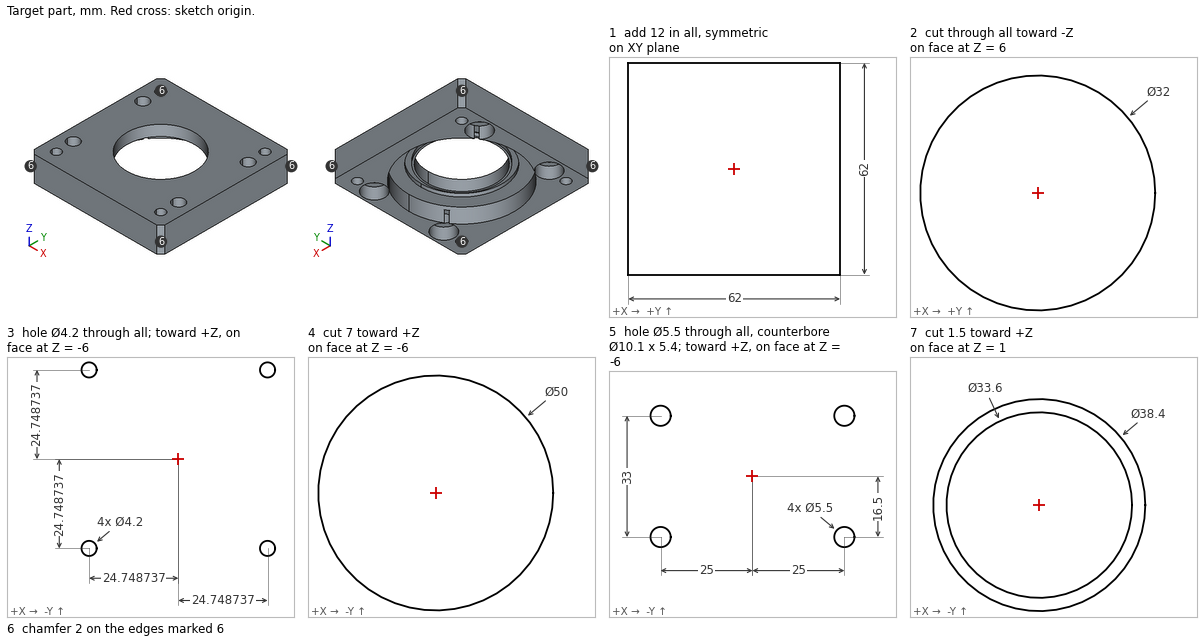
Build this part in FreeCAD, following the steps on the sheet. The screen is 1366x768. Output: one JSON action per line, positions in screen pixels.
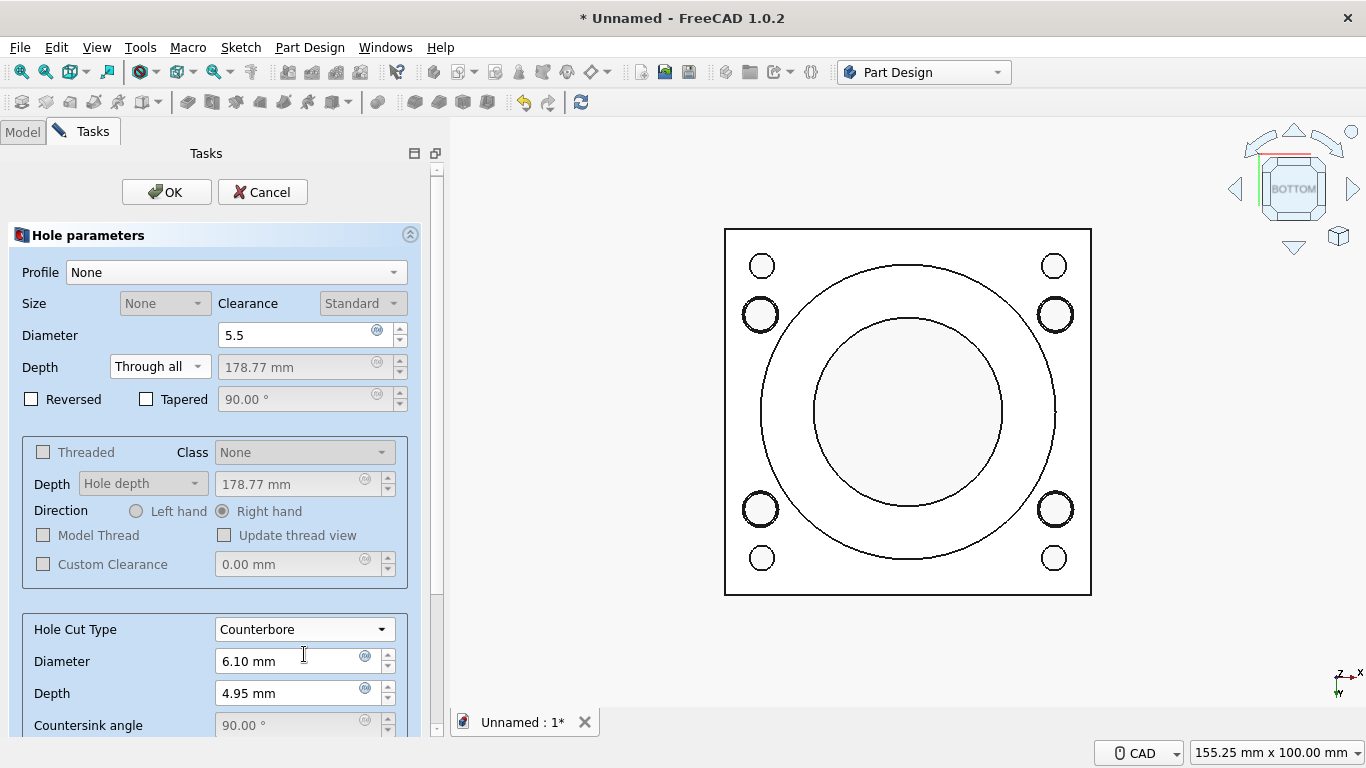
{"action": "triple_click", "coordinate": [298, 661]}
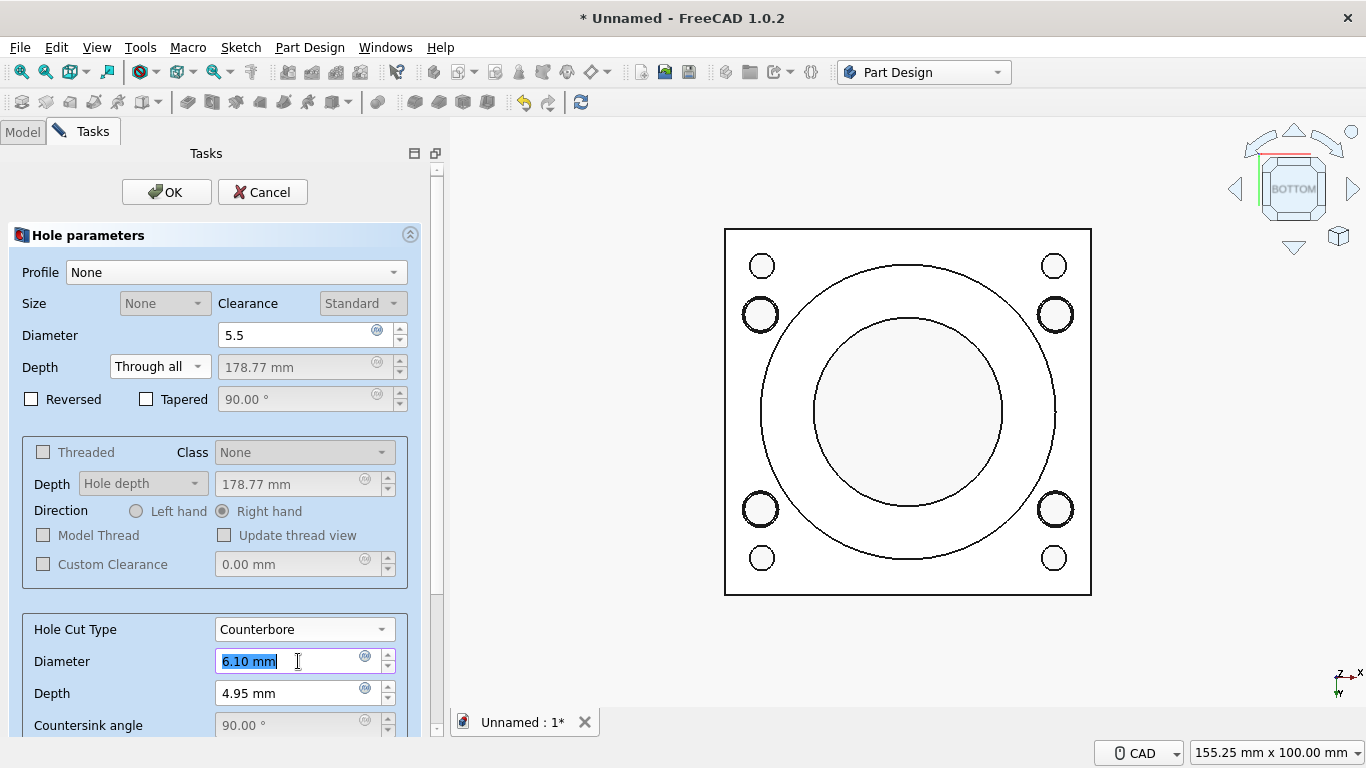
{"action": "type", "text": "10.1"}
{"action": "key", "text": "Tab"}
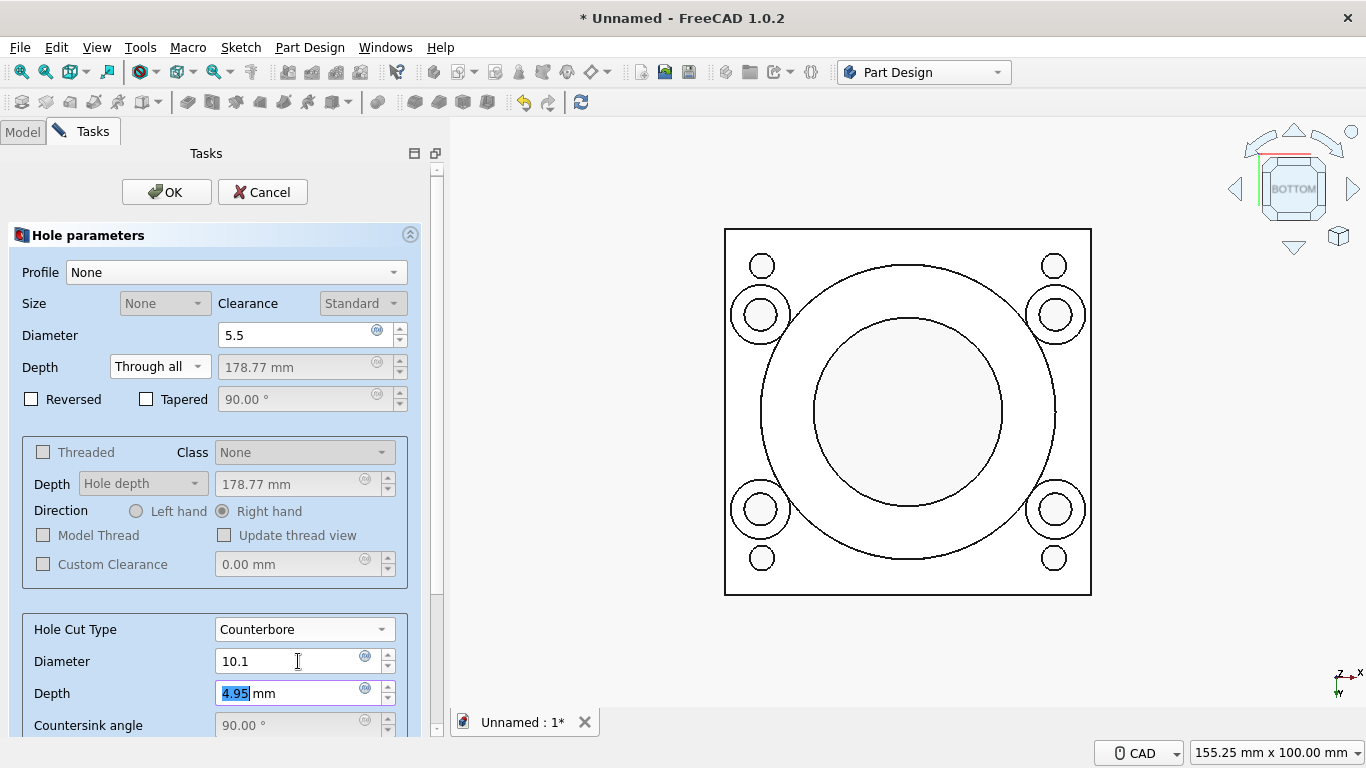
{"action": "type", "text": "5.4"}
{"action": "key", "text": "Tab"}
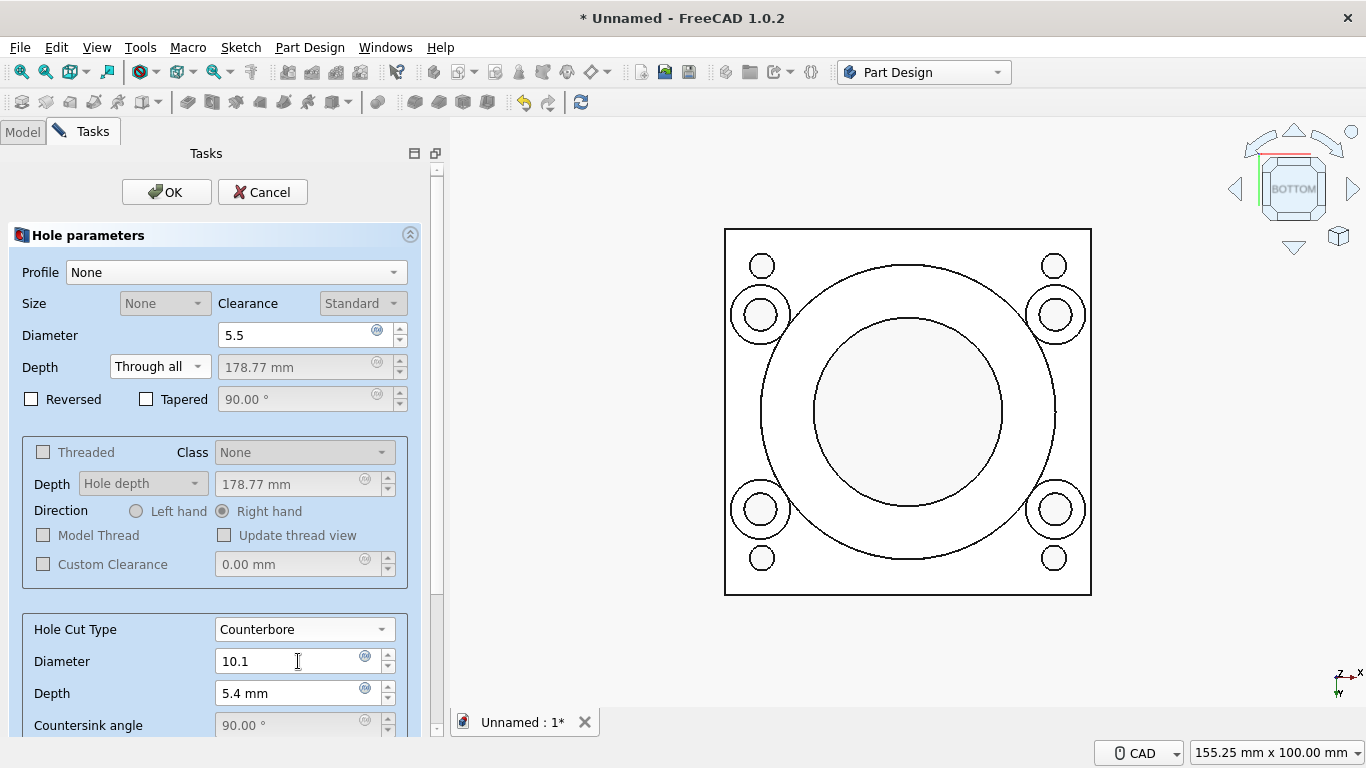
{"action": "left_click", "coordinate": [167, 192]}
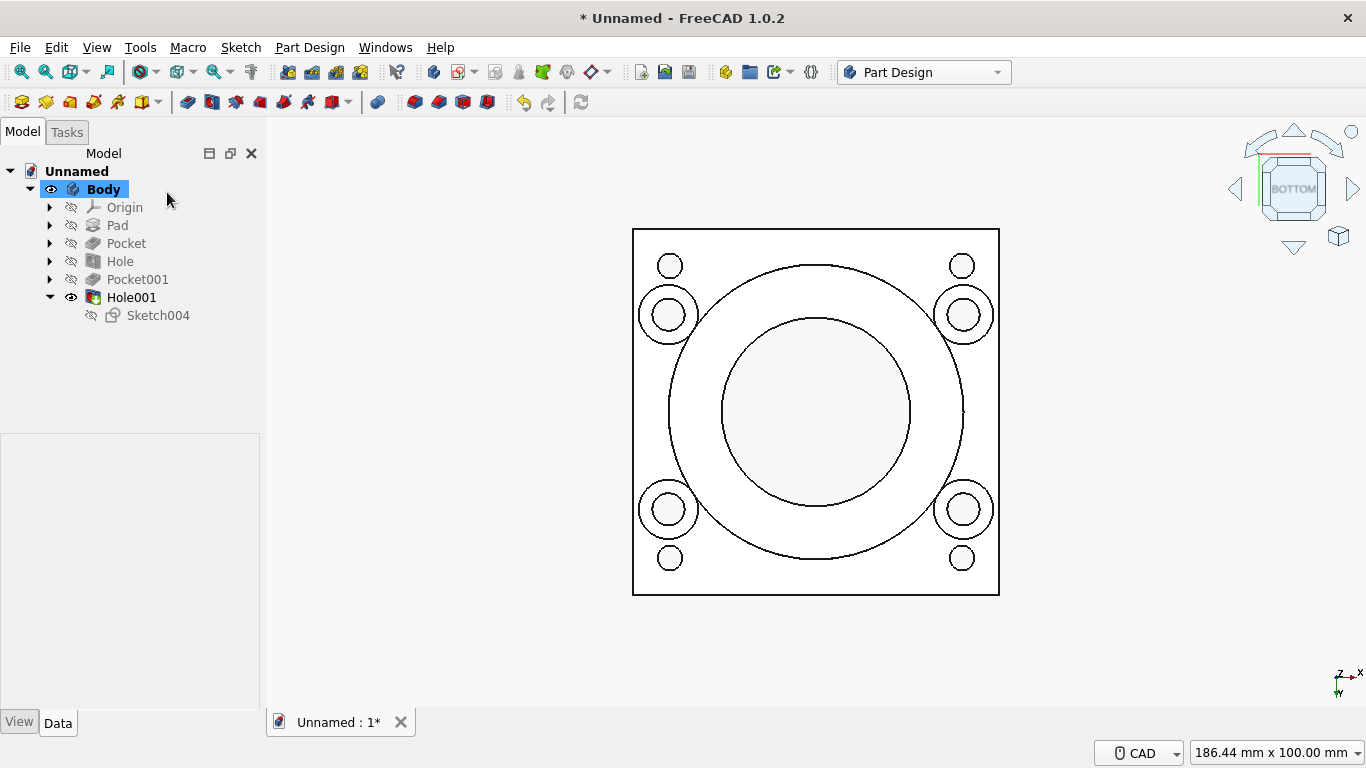
{"action": "key", "text": "0"}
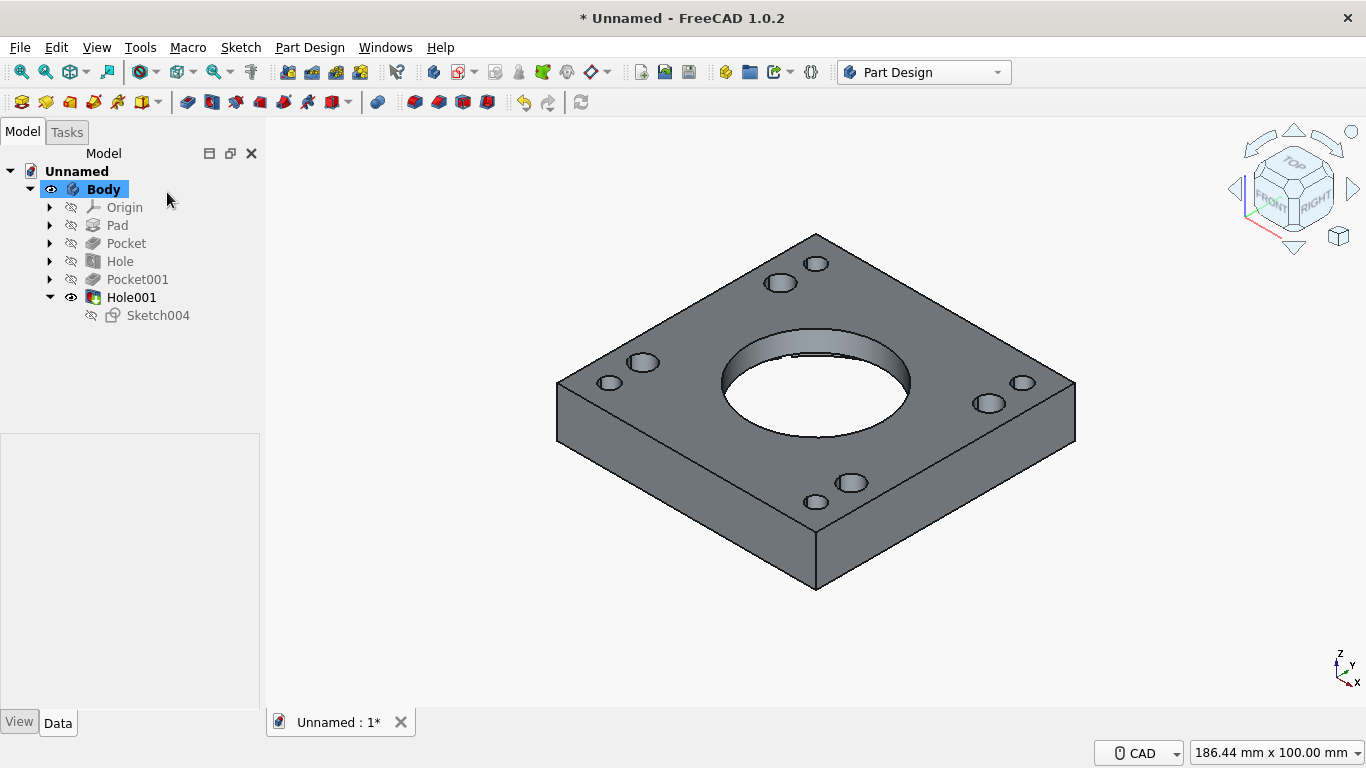
{"action": "left_click", "coordinate": [816, 560]}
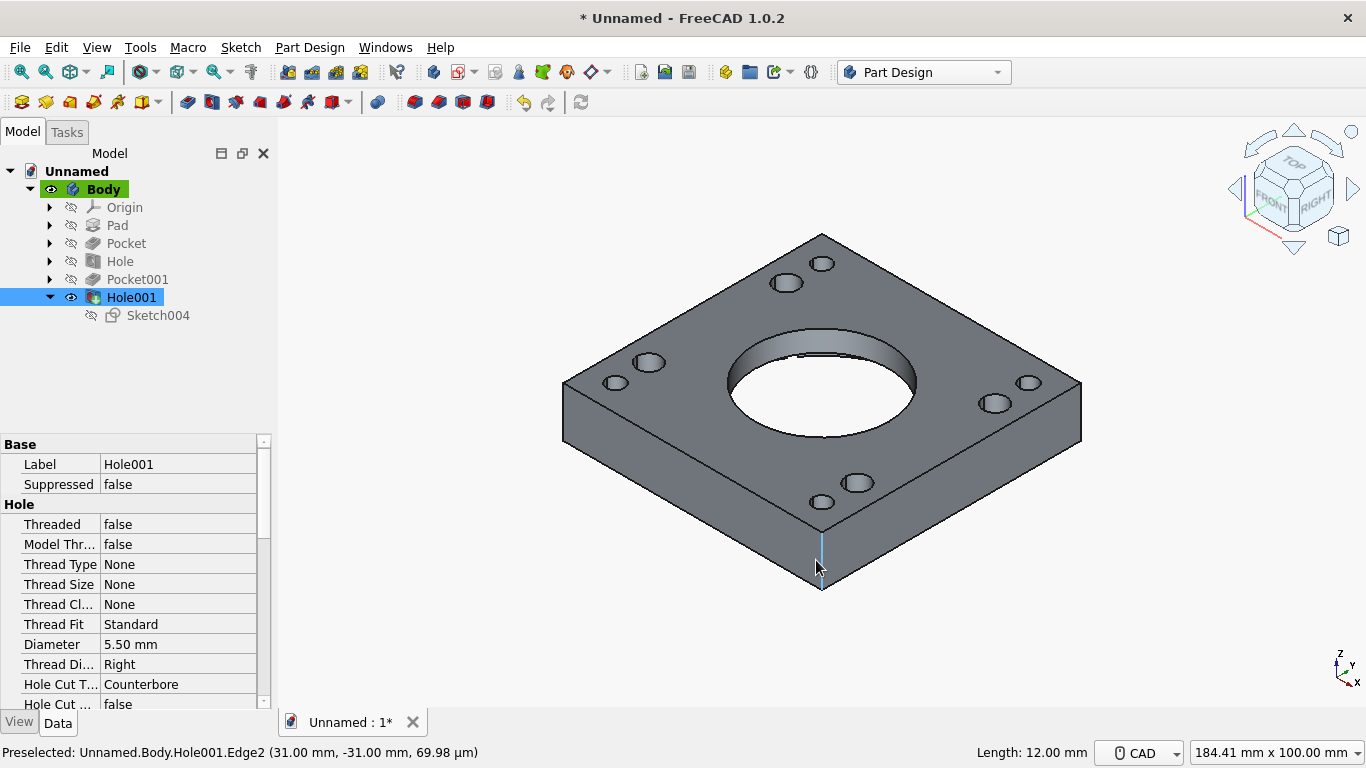
{"action": "key", "text": "2"}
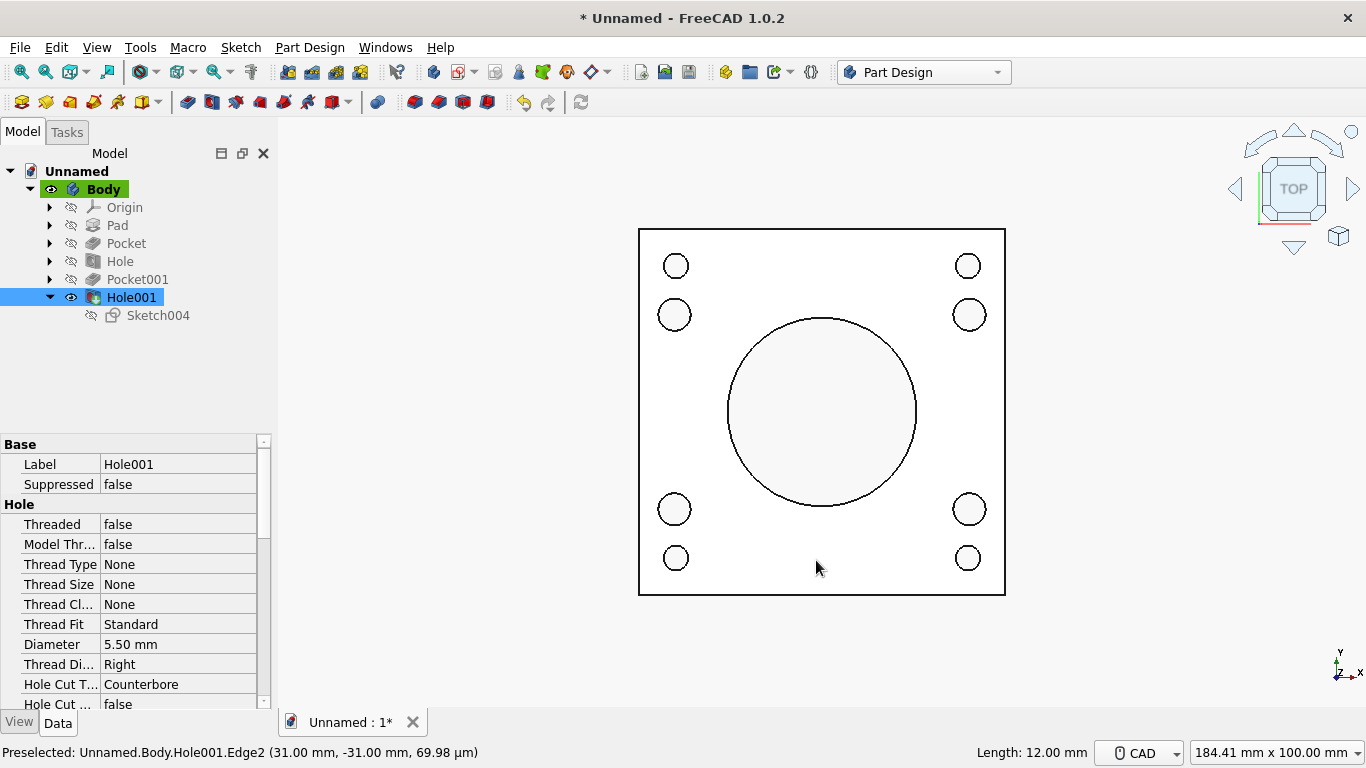
{"action": "key", "text": "1"}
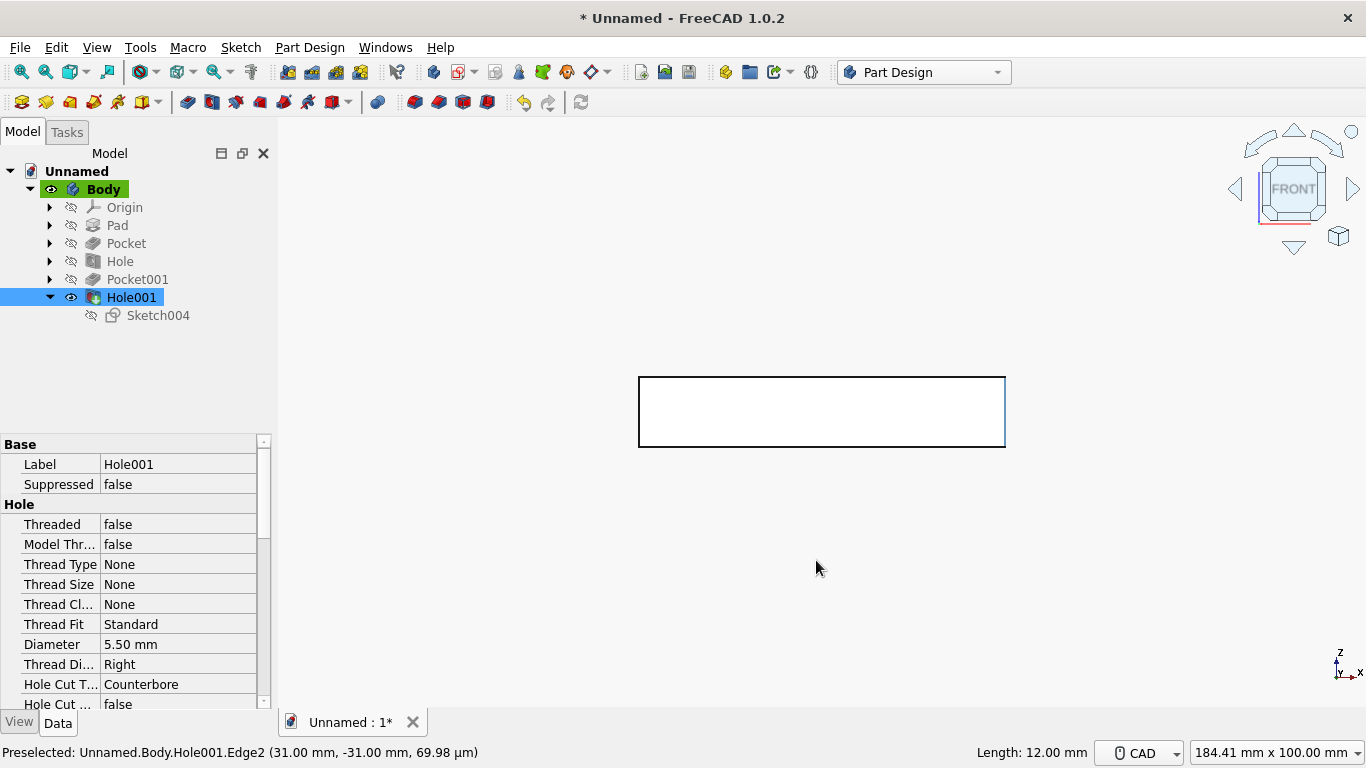
{"action": "left_click", "coordinate": [22, 72]}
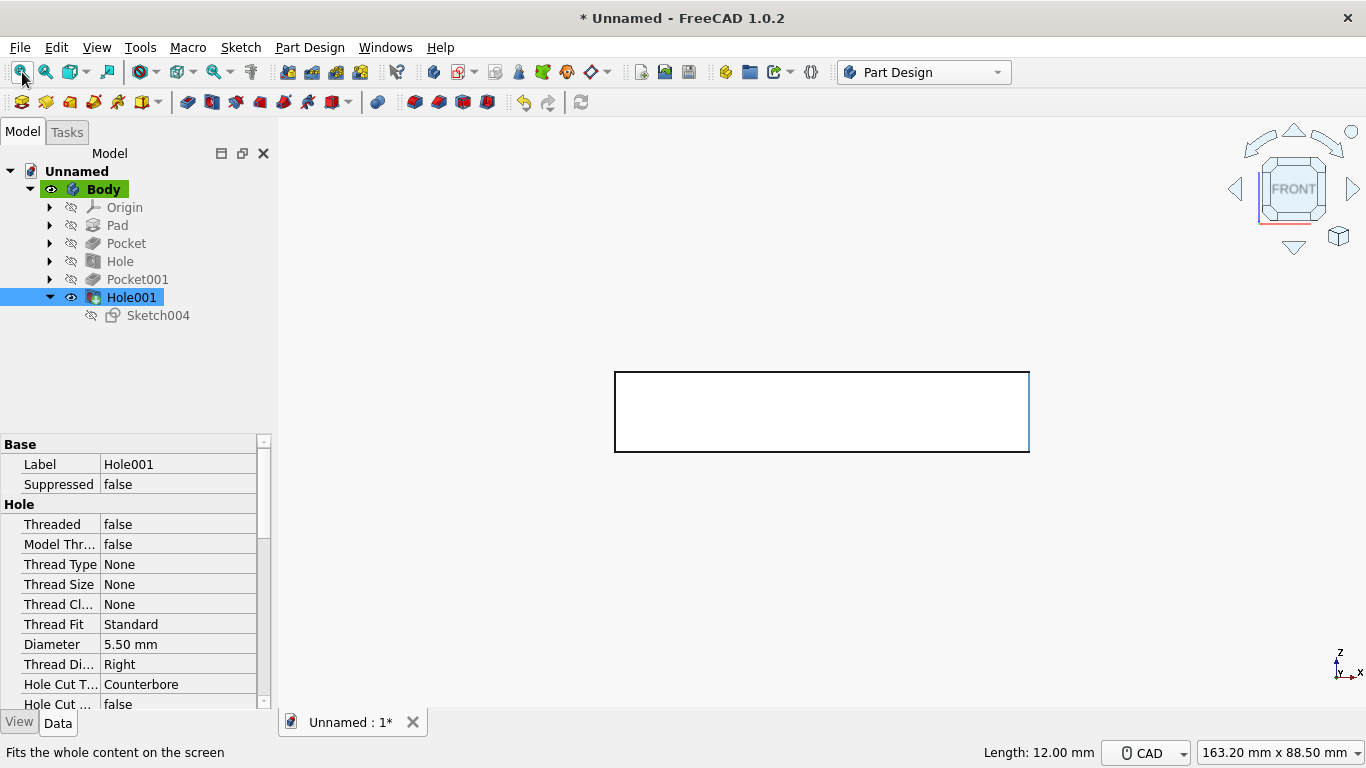
{"action": "left_click", "coordinate": [615, 411], "text": "ctrl"}